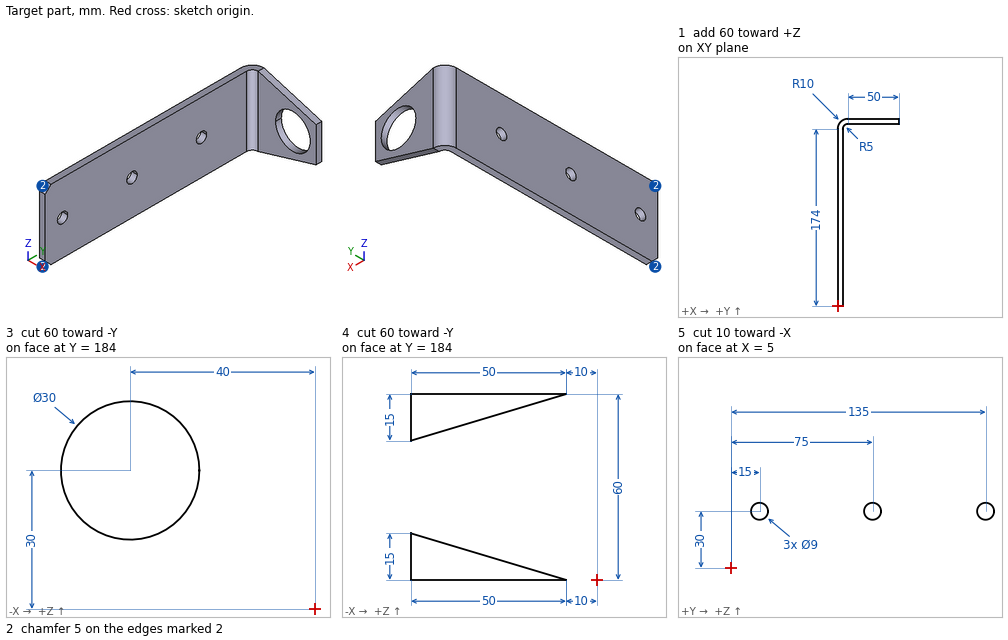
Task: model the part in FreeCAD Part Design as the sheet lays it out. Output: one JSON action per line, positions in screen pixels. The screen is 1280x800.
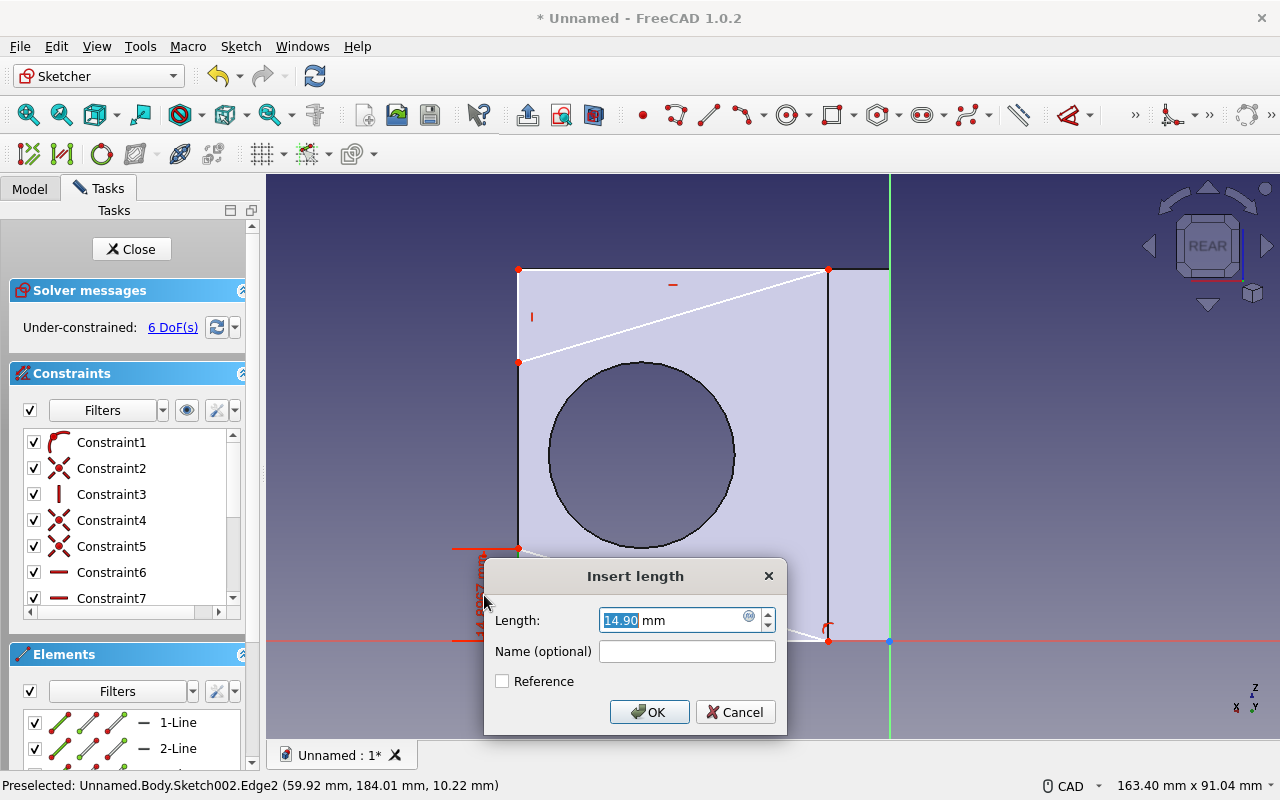
{"action": "type", "text": "15"}
{"action": "key", "text": "Return"}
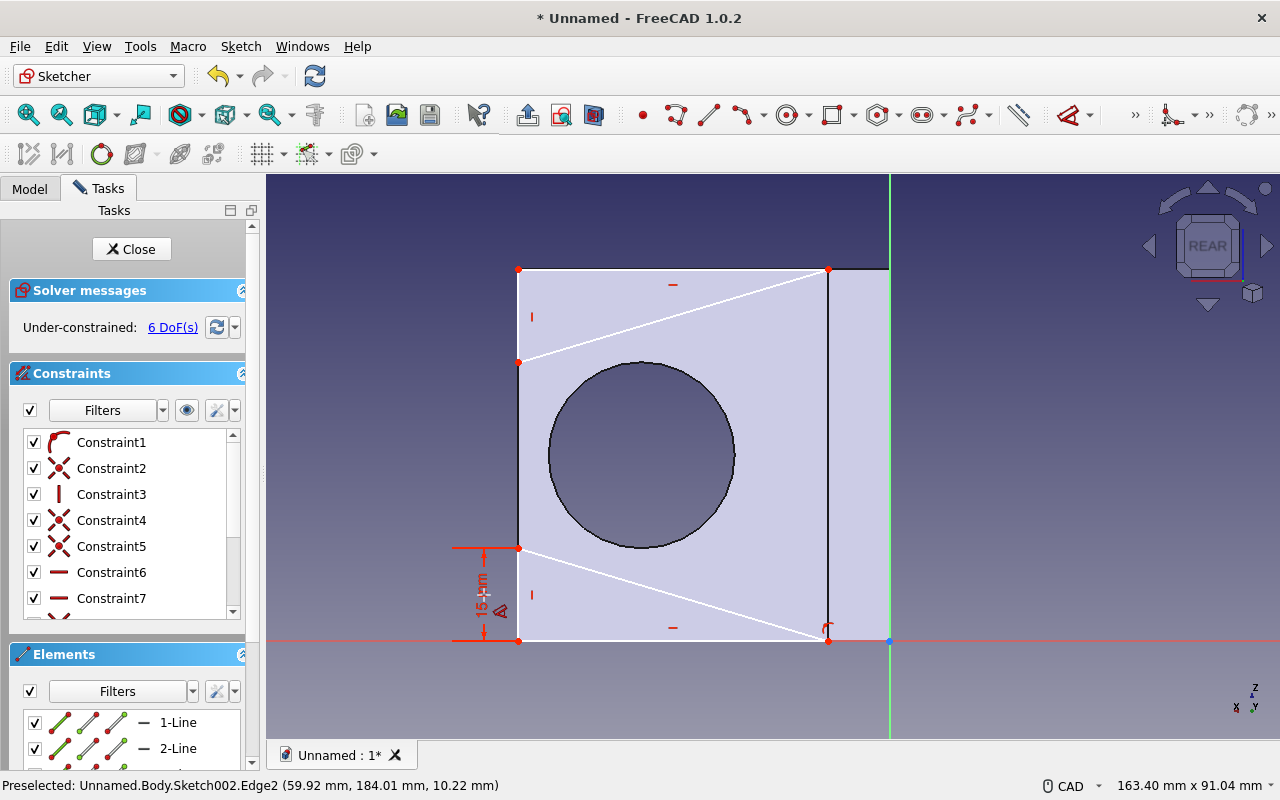
{"action": "left_click", "coordinate": [611, 641]}
{"action": "left_click", "coordinate": [673, 675]}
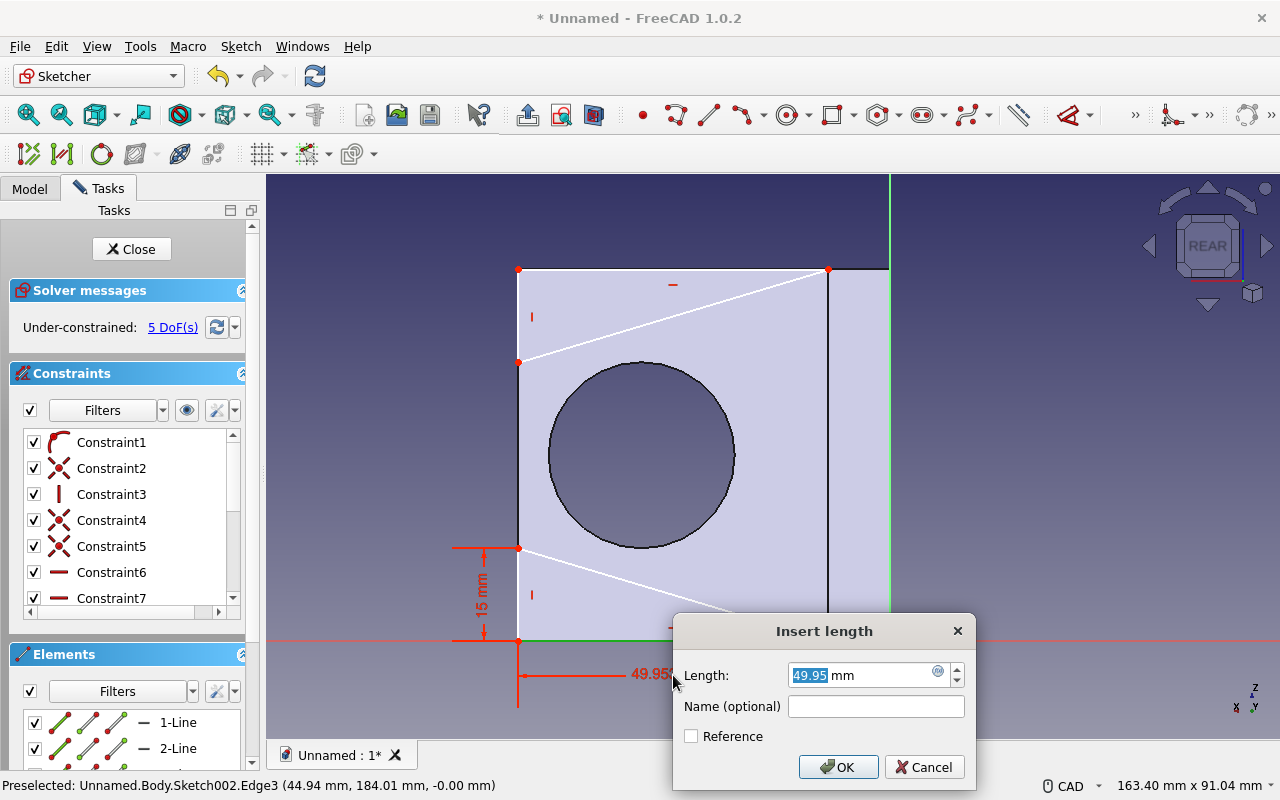
{"action": "type", "text": "50"}
{"action": "key", "text": "Return"}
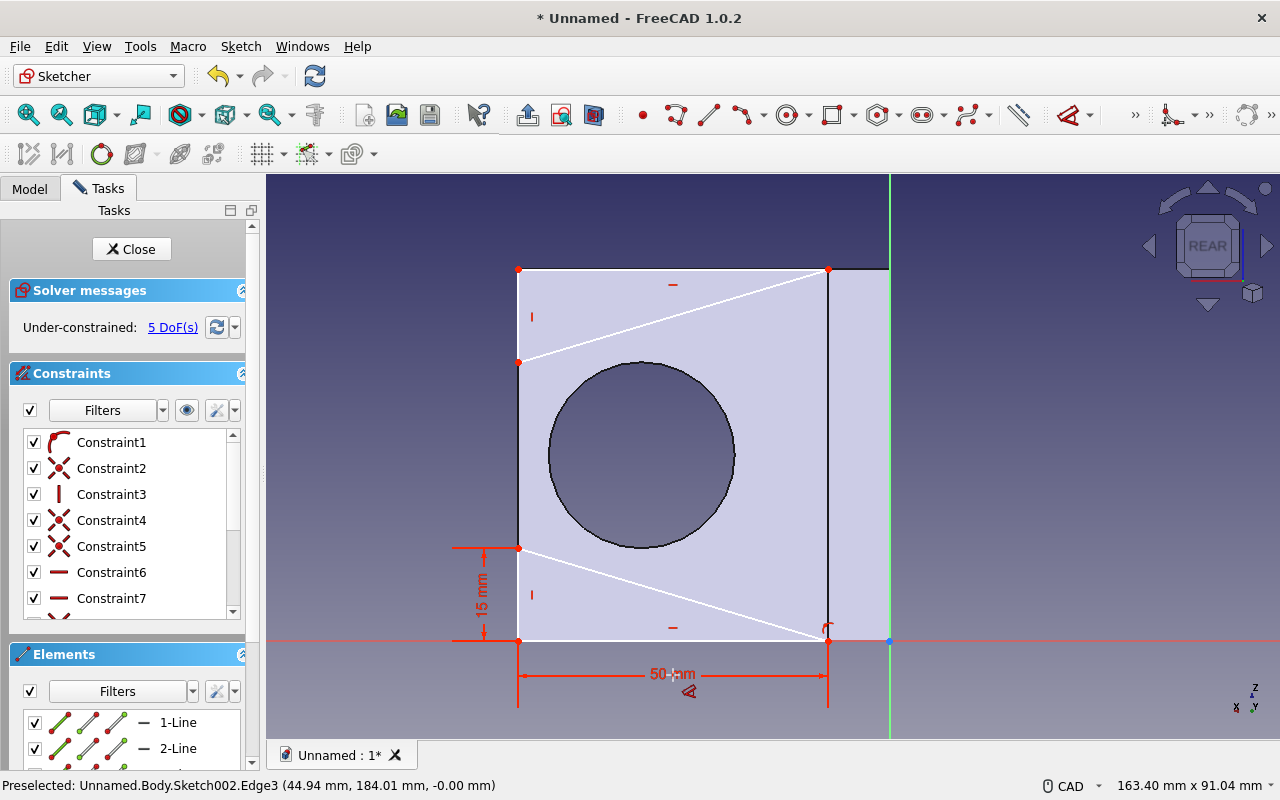
{"action": "left_click", "coordinate": [735, 270]}
{"action": "left_click", "coordinate": [673, 236]}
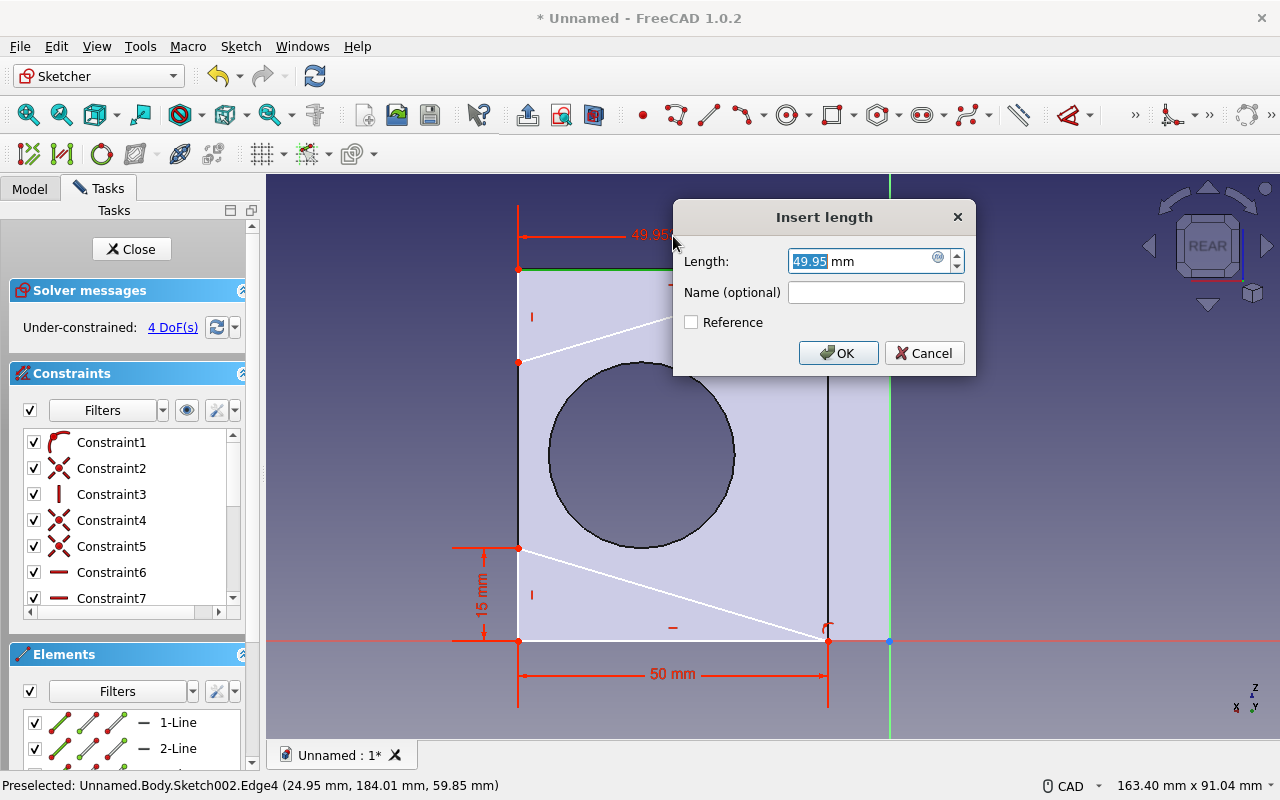
{"action": "type", "text": "50"}
{"action": "key", "text": "Return"}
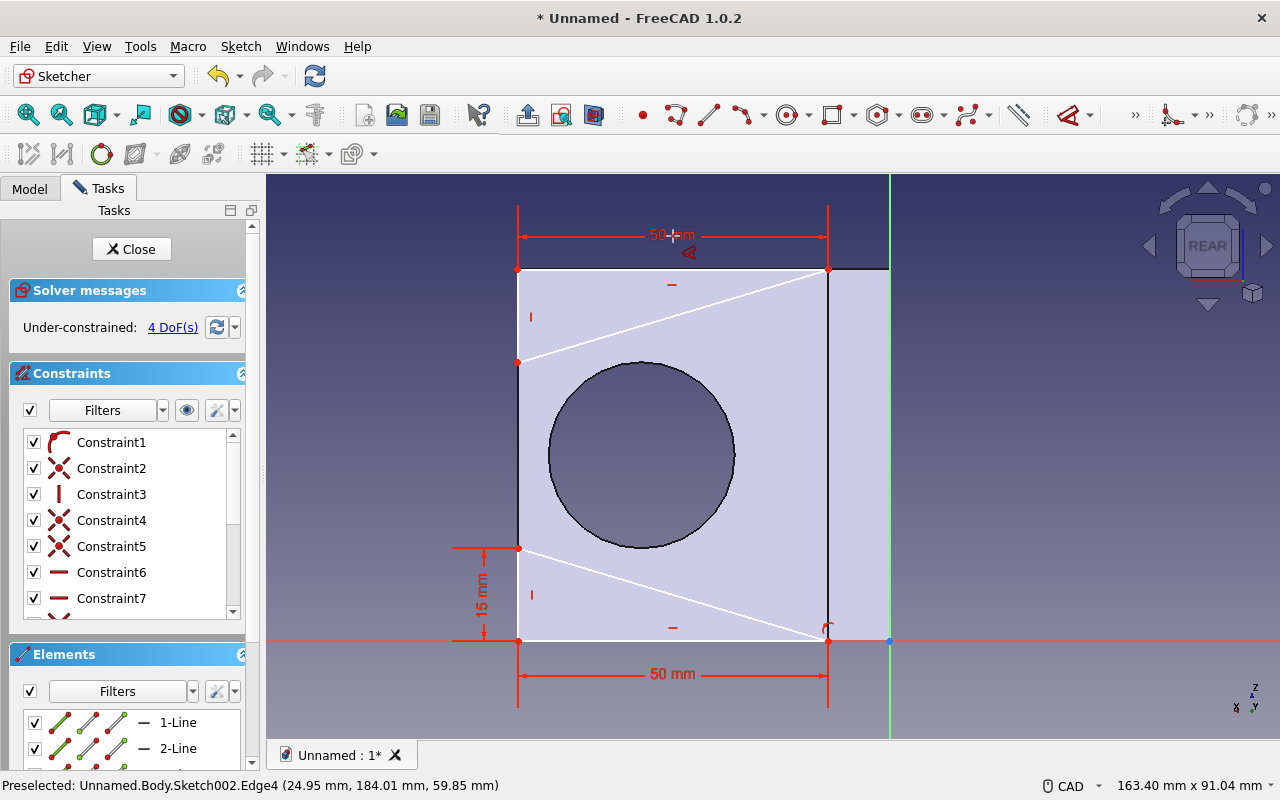
{"action": "left_click", "coordinate": [518, 298]}
{"action": "left_click", "coordinate": [484, 316]}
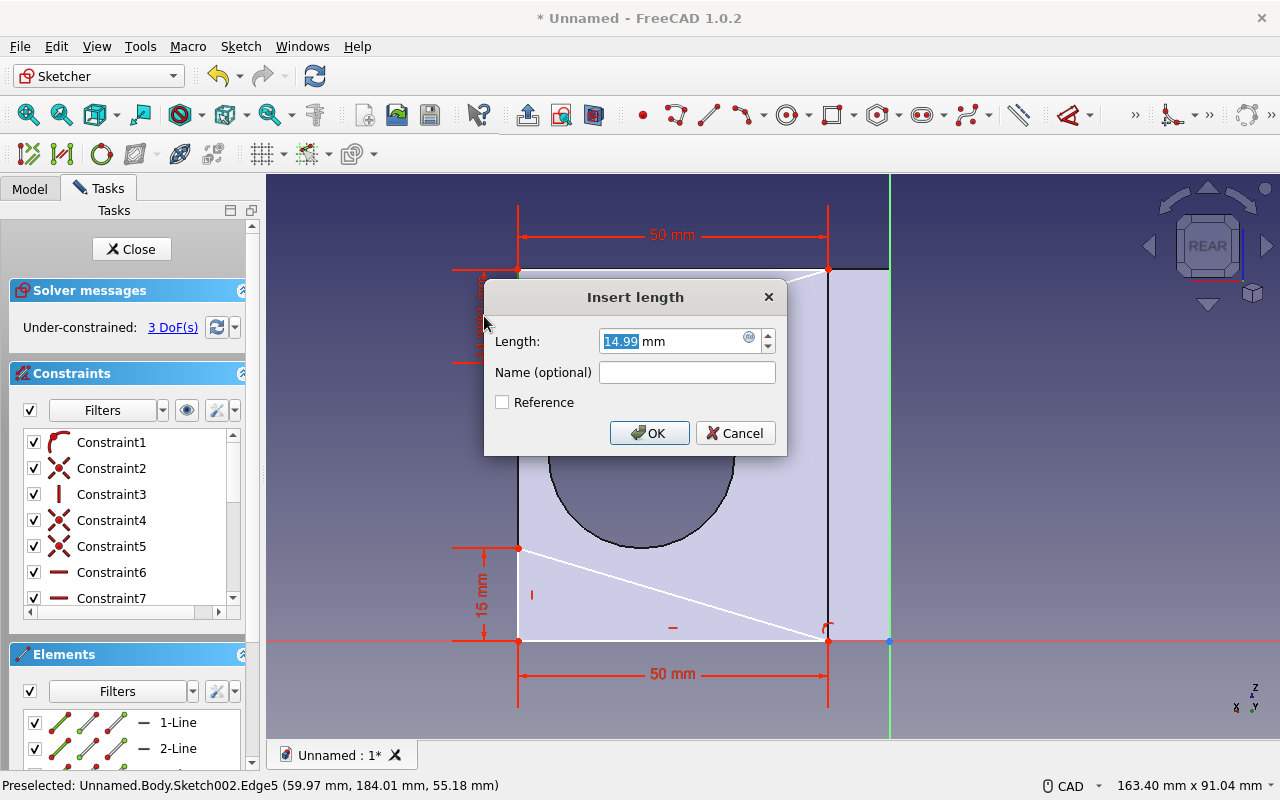
{"action": "type", "text": "15"}
{"action": "key", "text": "Return"}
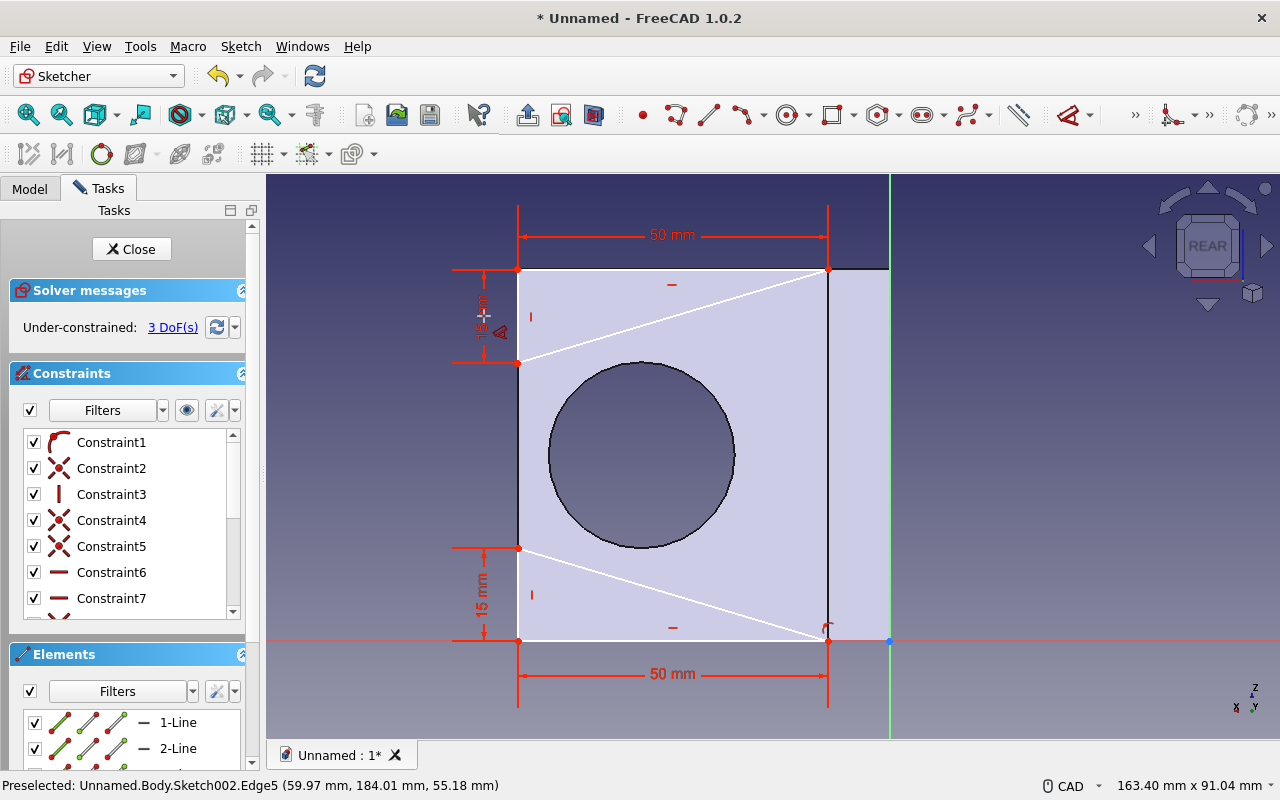
{"action": "left_click", "coordinate": [828, 641]}
{"action": "left_click", "coordinate": [859, 675]}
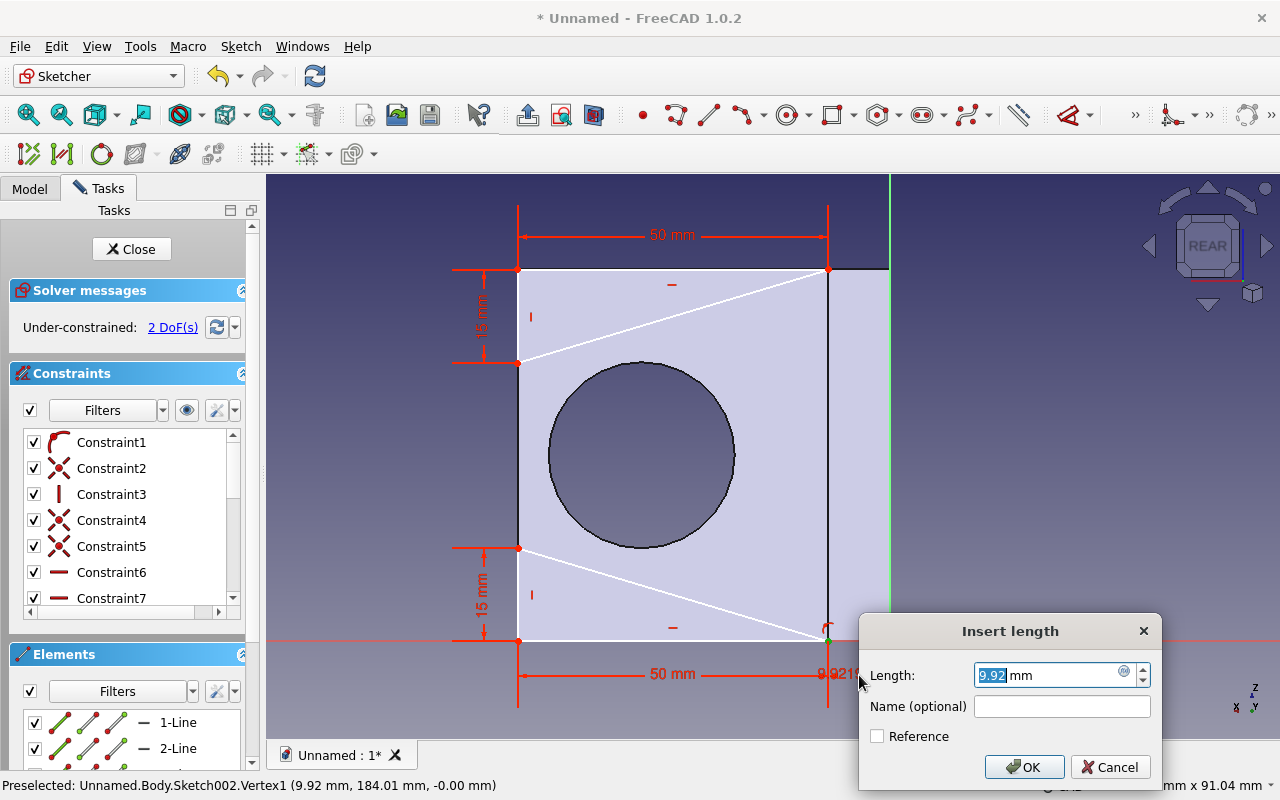
{"action": "type", "text": "10"}
{"action": "key", "text": "Return"}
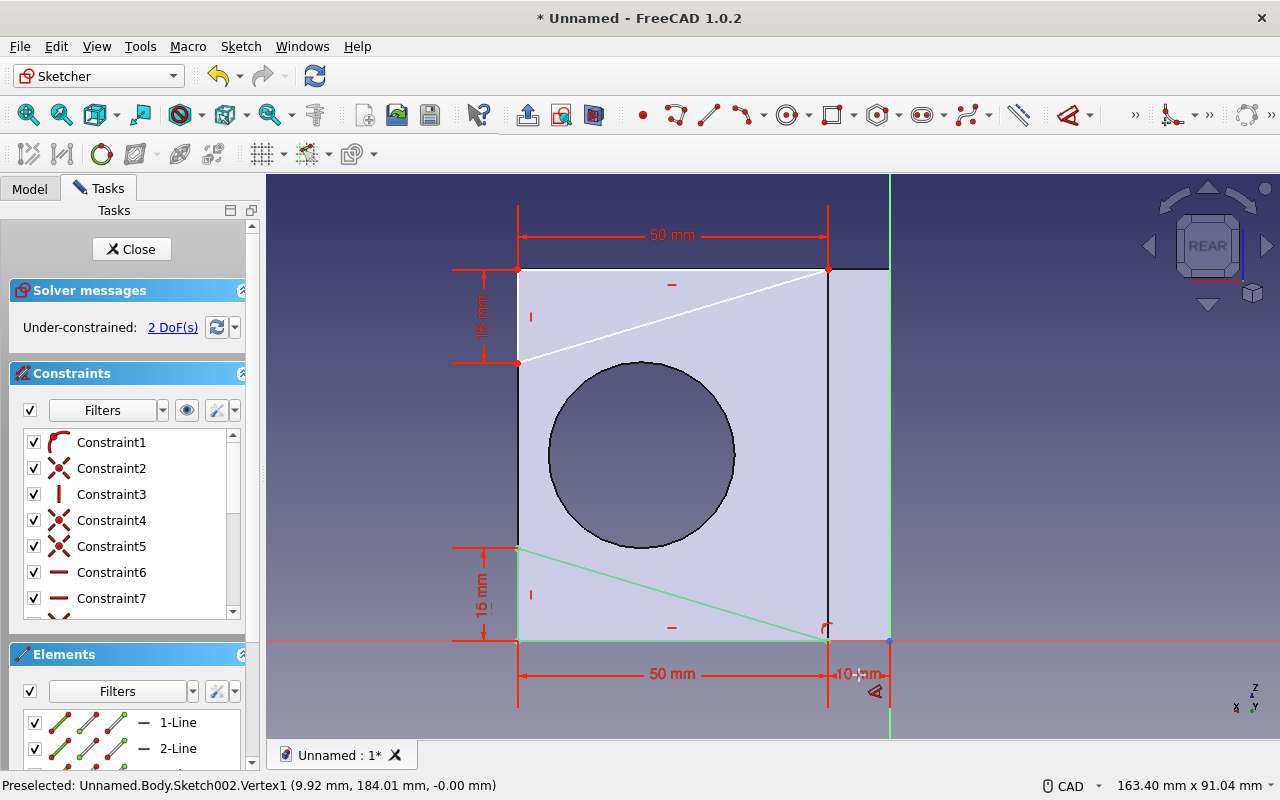
{"action": "left_click", "coordinate": [828, 270]}
{"action": "left_click", "coordinate": [859, 236]}